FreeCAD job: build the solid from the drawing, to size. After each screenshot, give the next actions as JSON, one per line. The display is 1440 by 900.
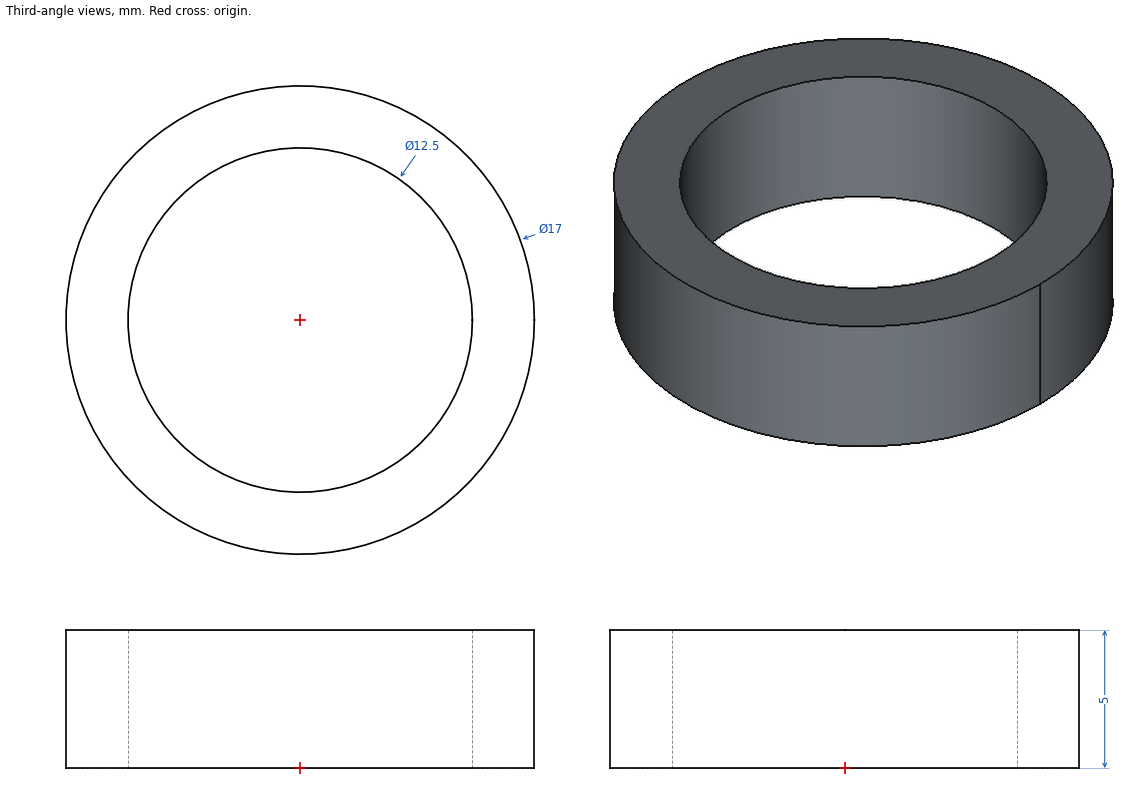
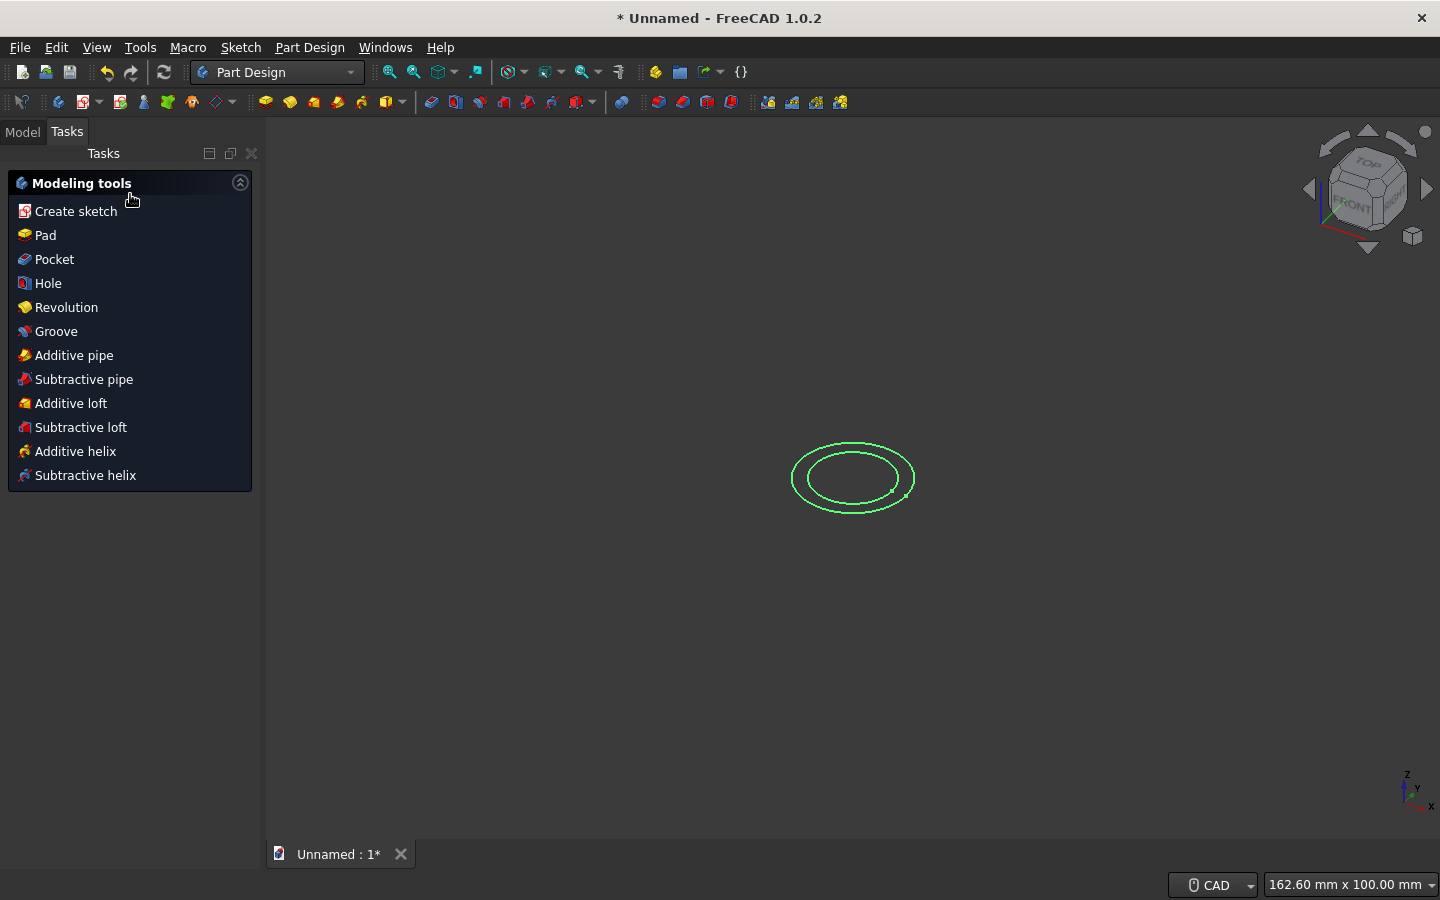
{"action": "left_click", "coordinate": [266, 102]}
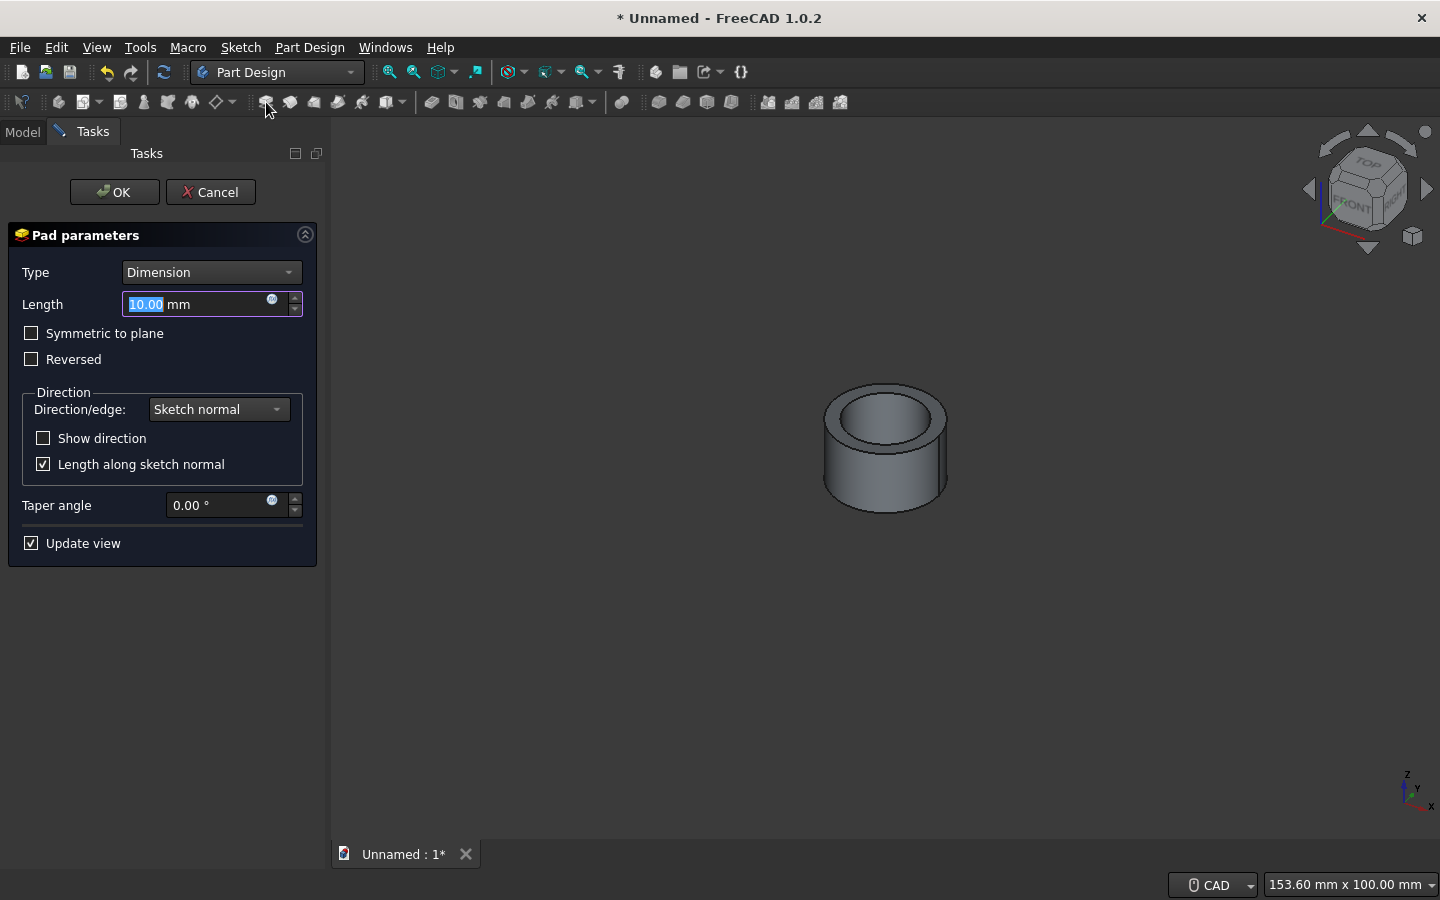
{"action": "type", "text": "5"}
{"action": "key", "text": "Tab"}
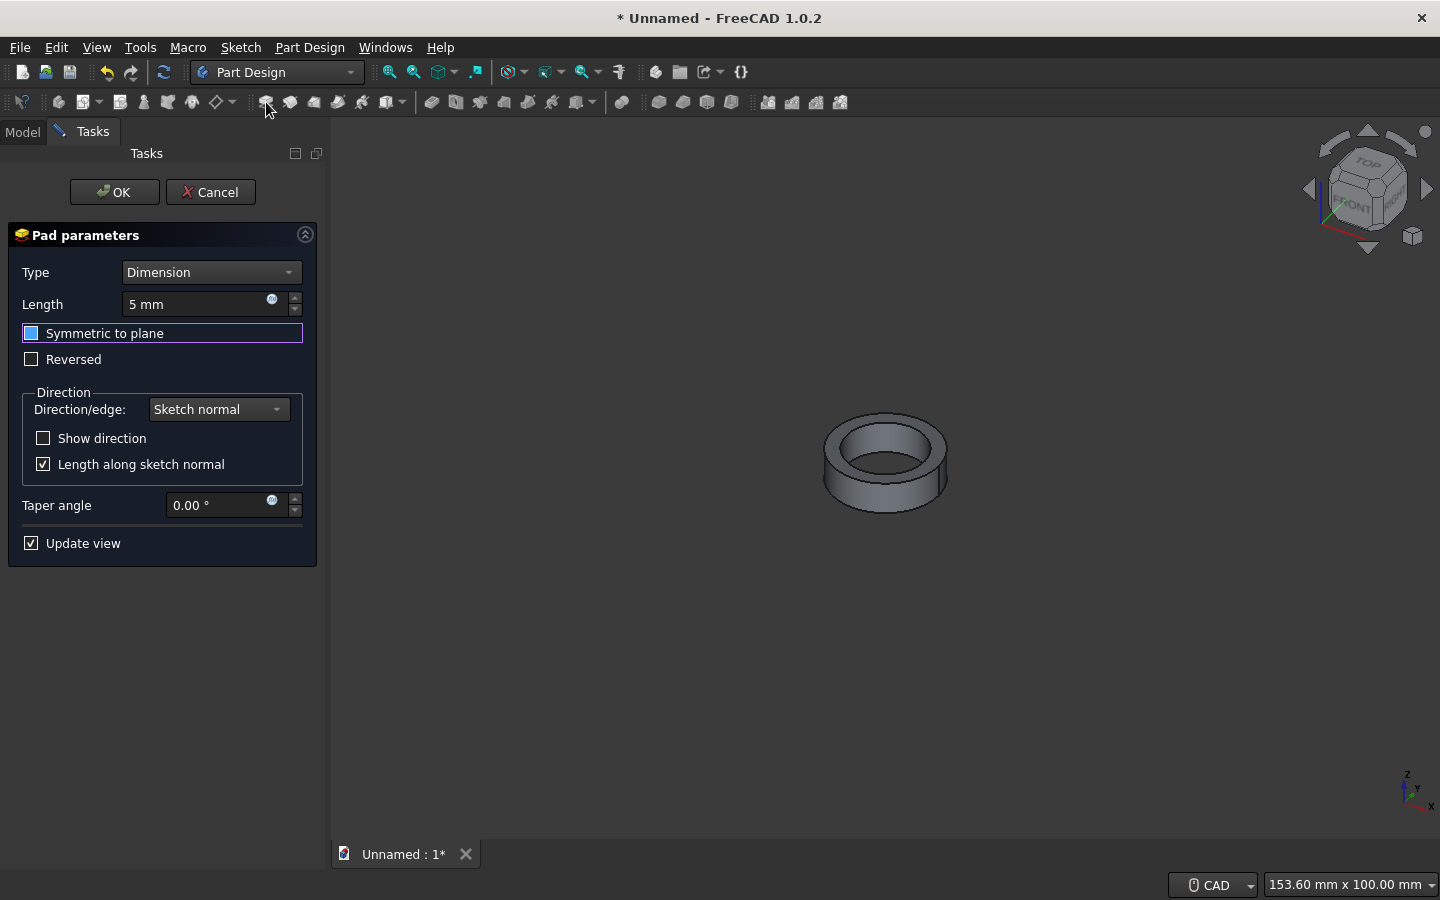
{"action": "left_click", "coordinate": [115, 192]}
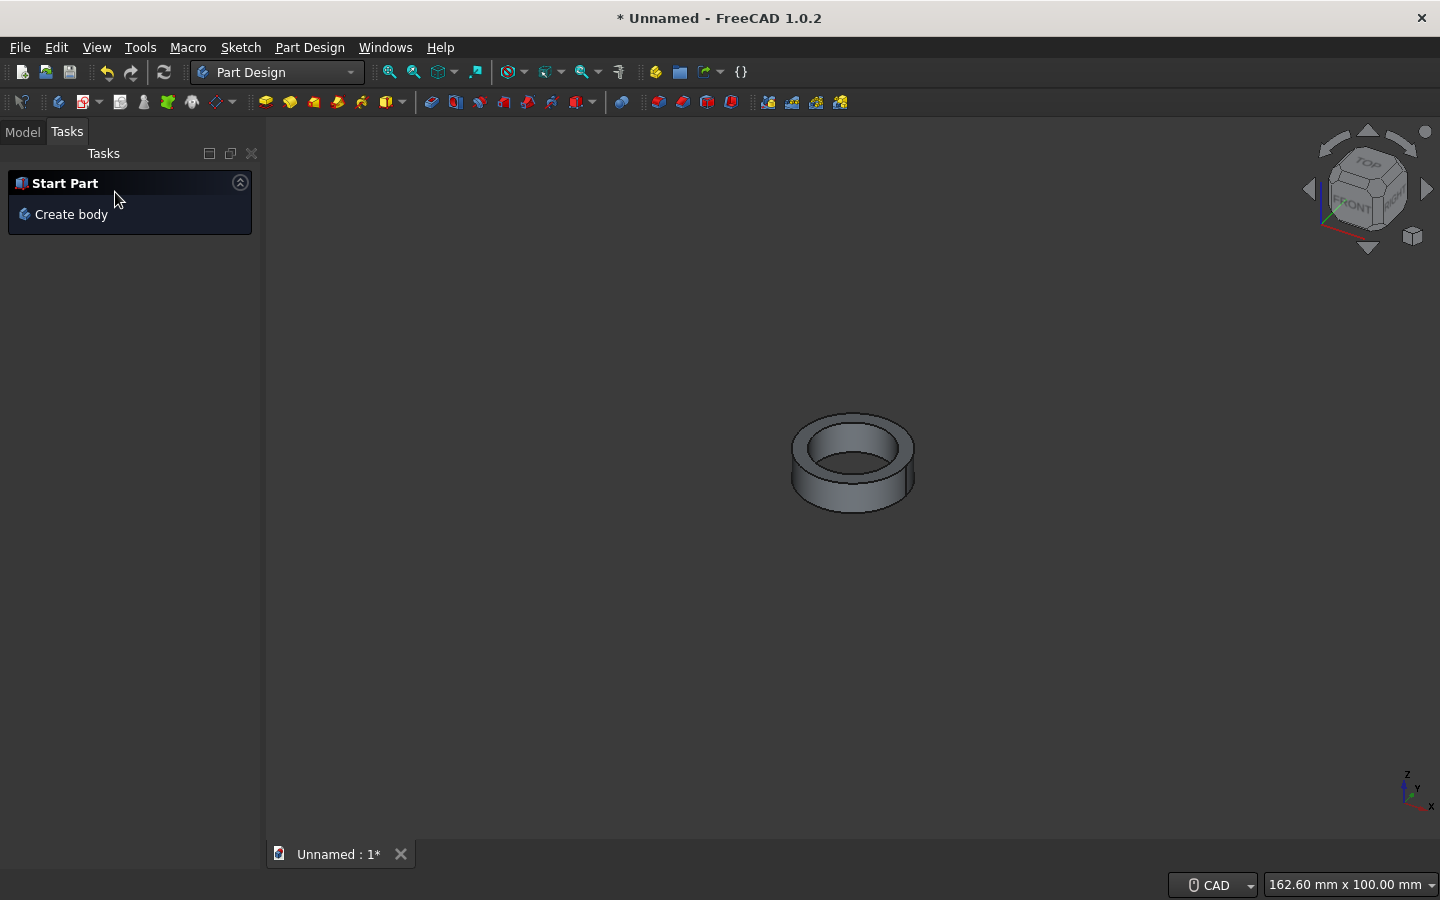
{"action": "key", "text": "0"}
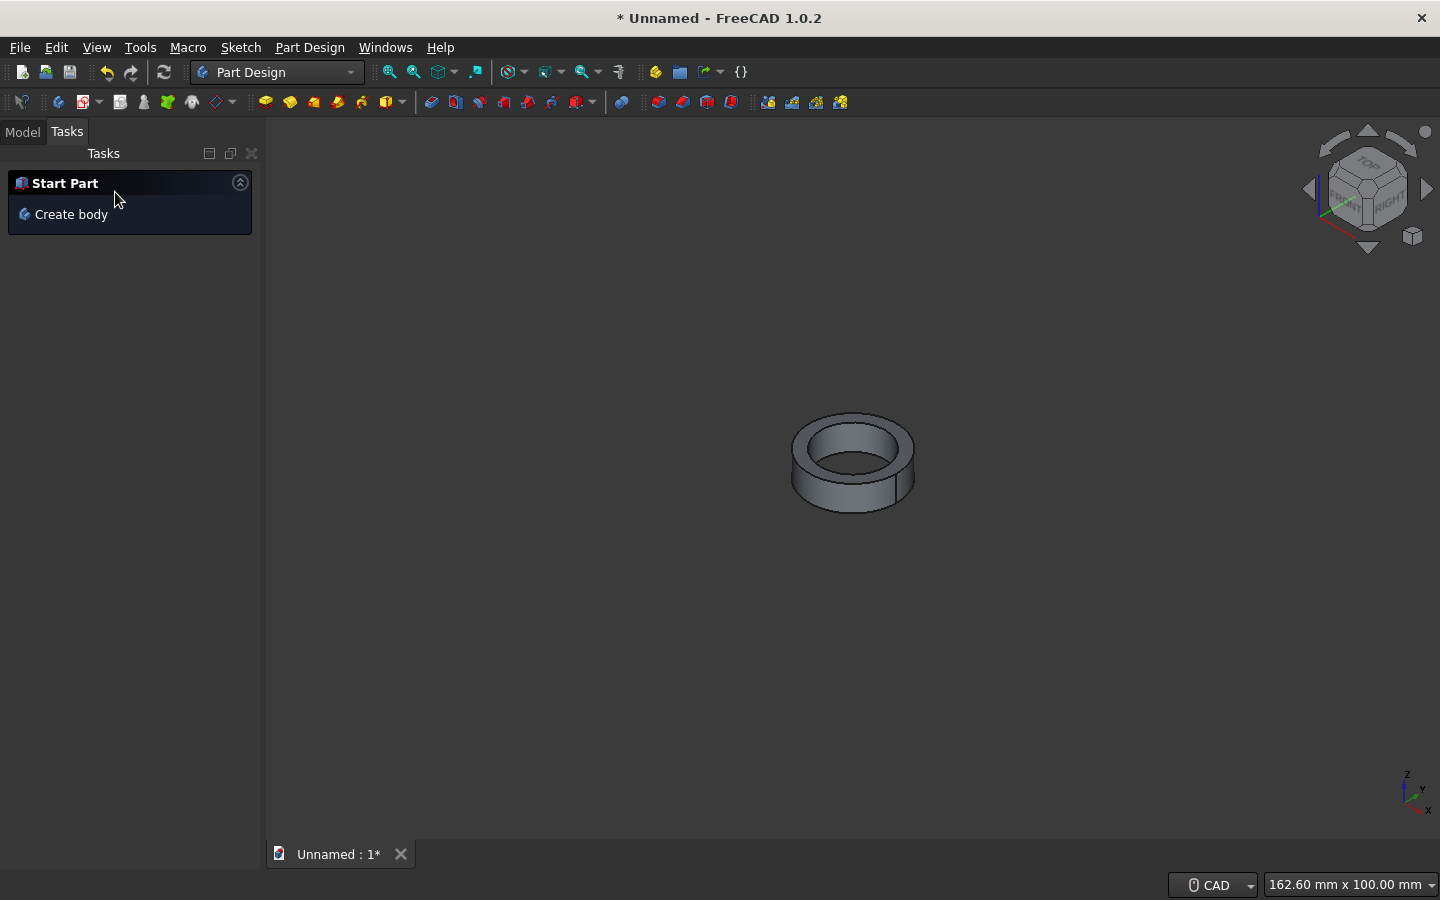
{"action": "key", "text": "v f"}